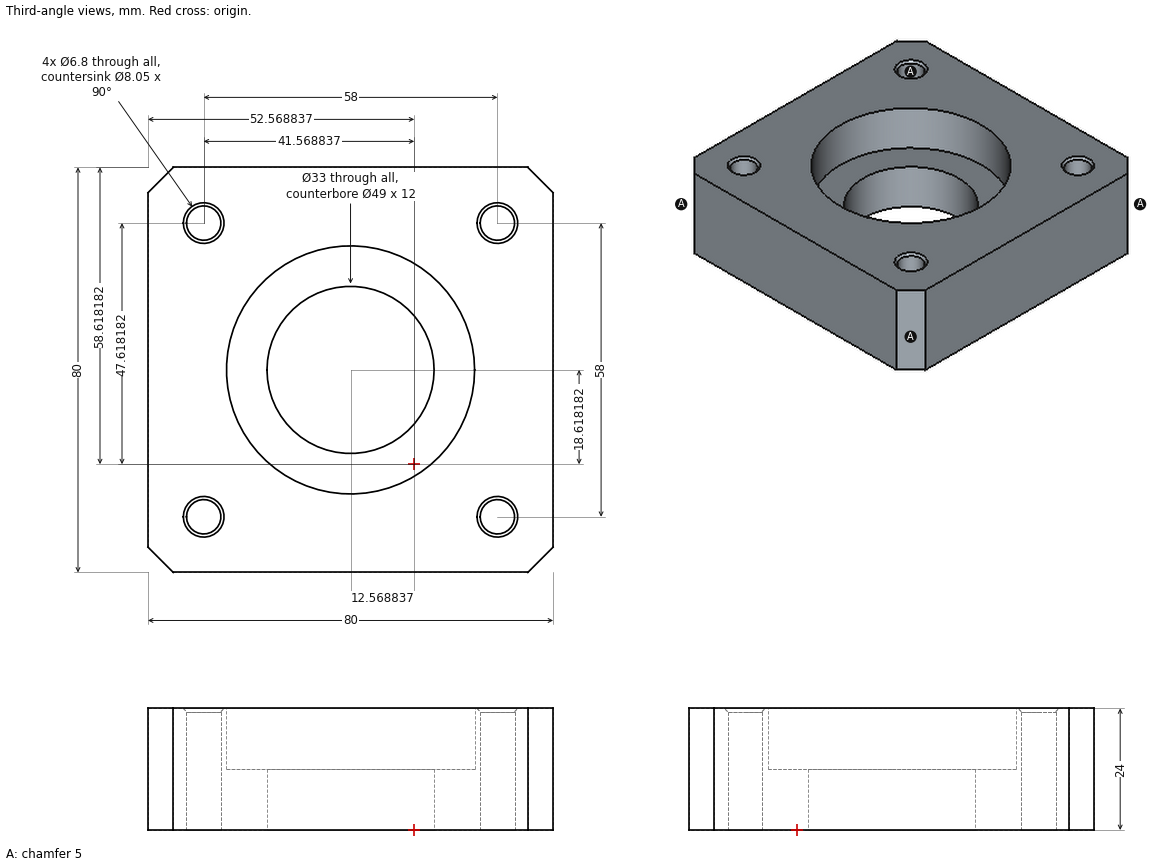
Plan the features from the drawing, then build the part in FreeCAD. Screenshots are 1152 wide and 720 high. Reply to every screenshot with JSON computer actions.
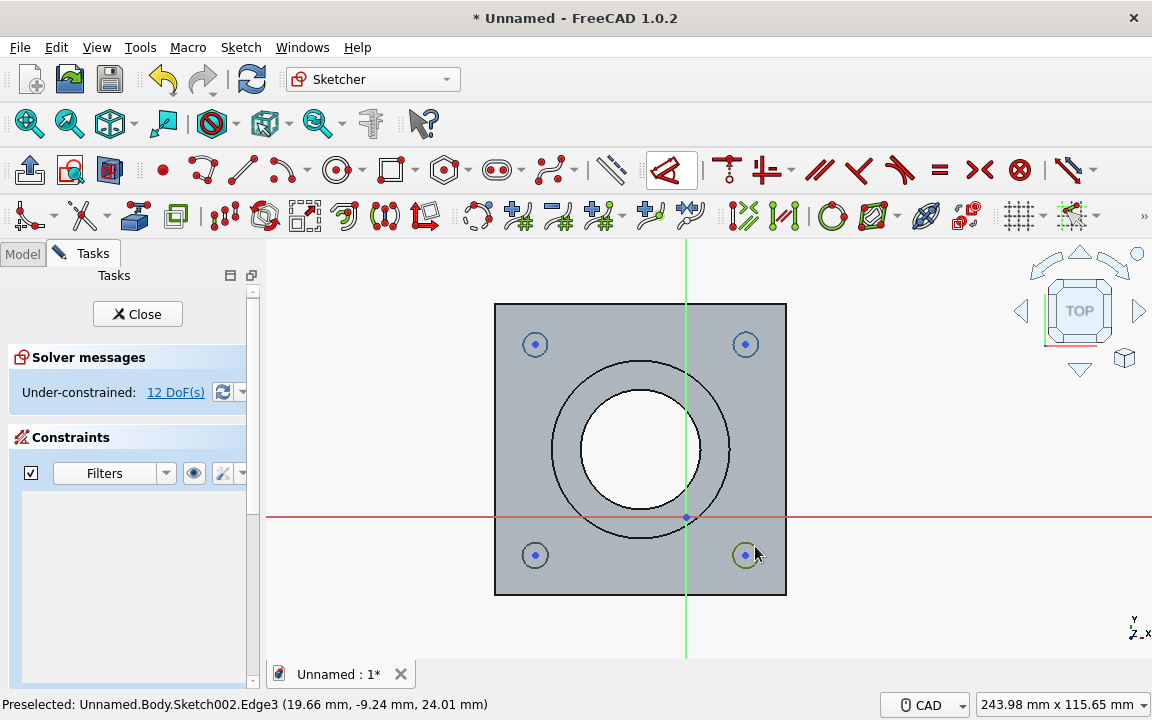
{"action": "left_click", "coordinate": [544, 546]}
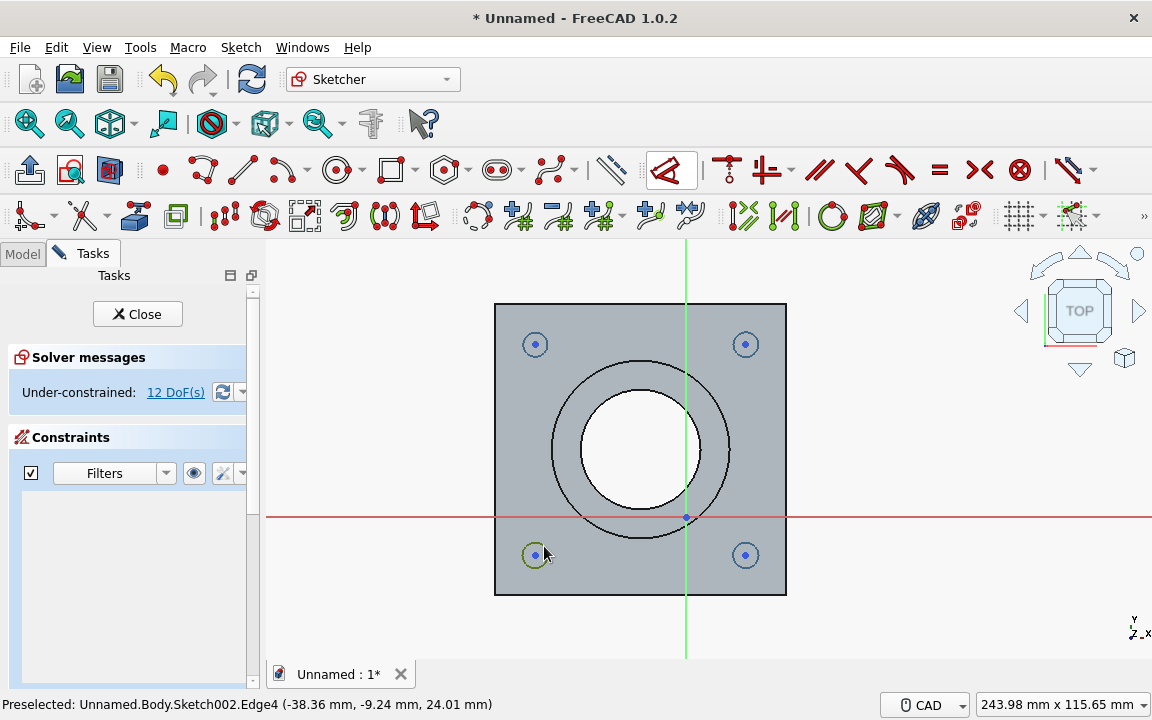
{"action": "key", "text": "e"}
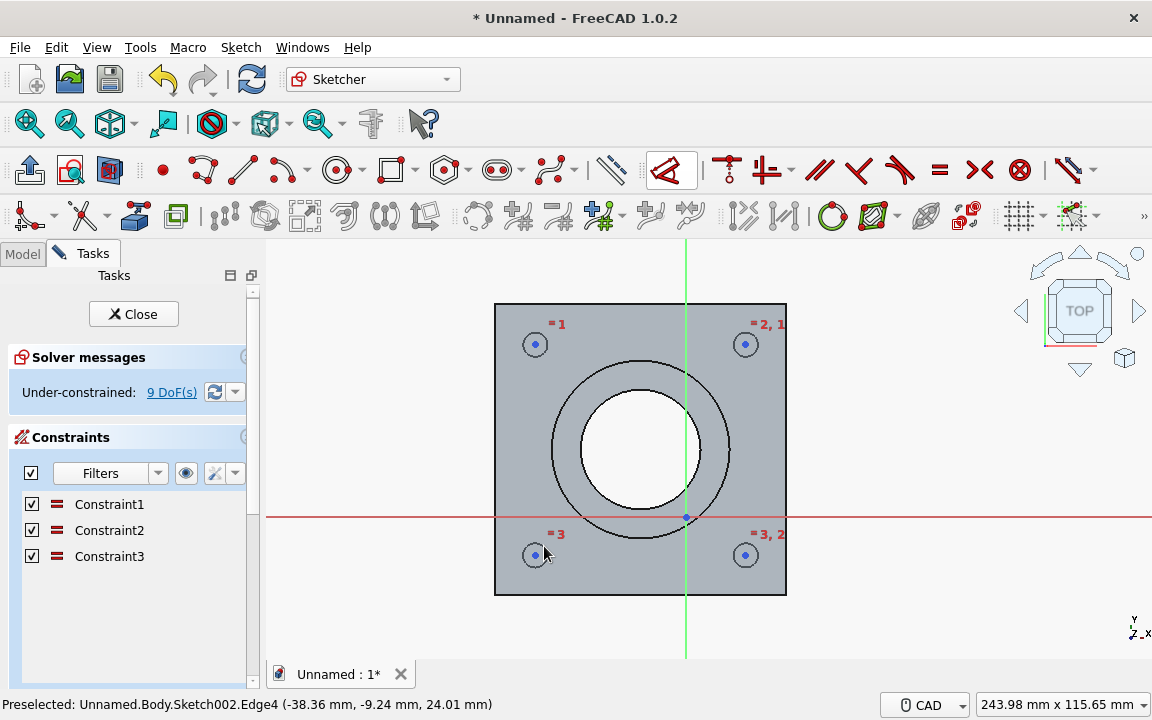
{"action": "scroll", "coordinate": [544, 336], "scroll_direction": "up", "scroll_amount": 3}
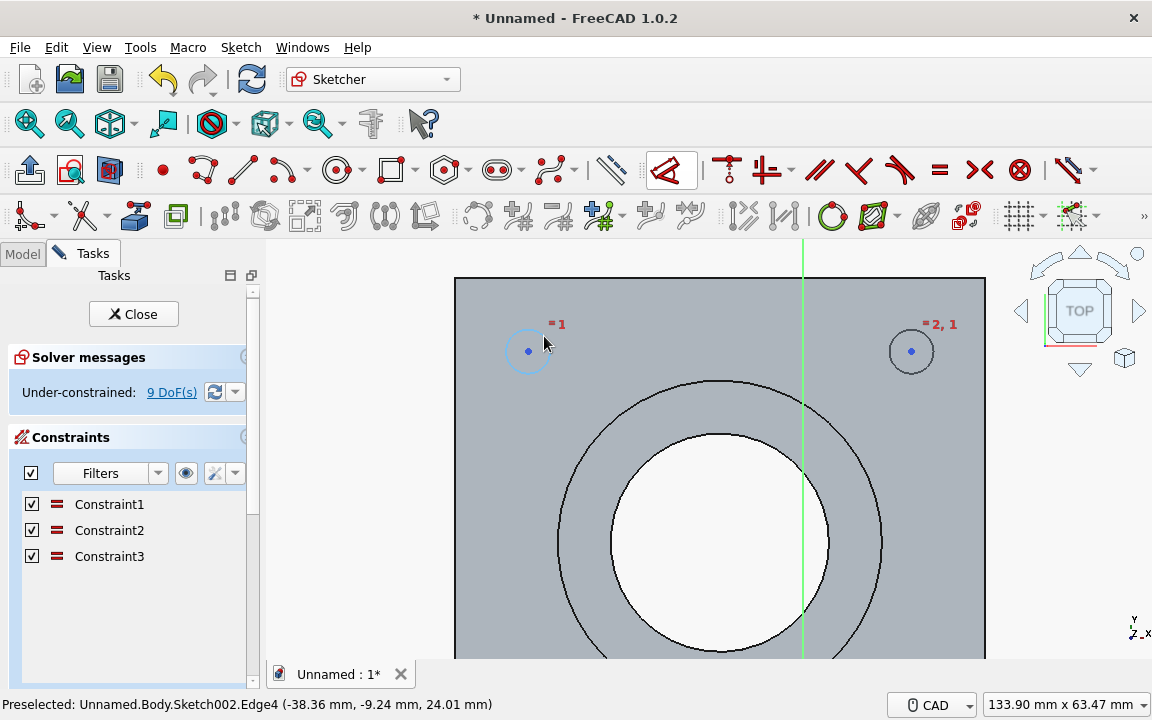
{"action": "left_click", "coordinate": [544, 336]}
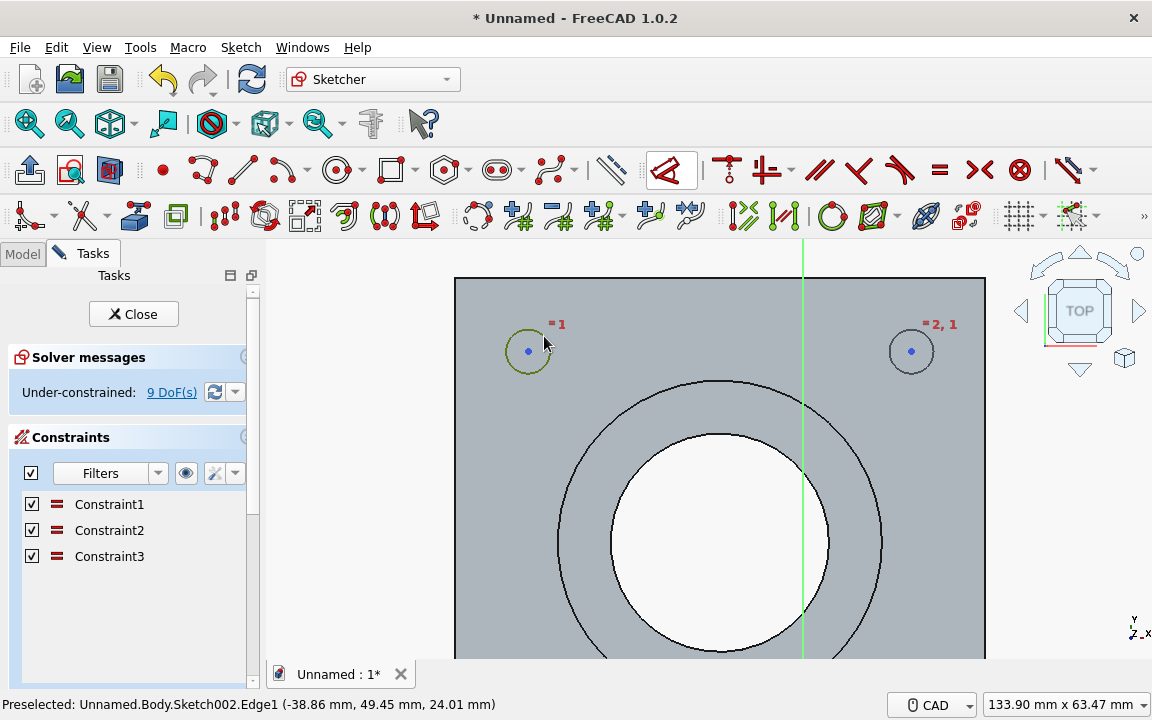
{"action": "key", "text": "k o"}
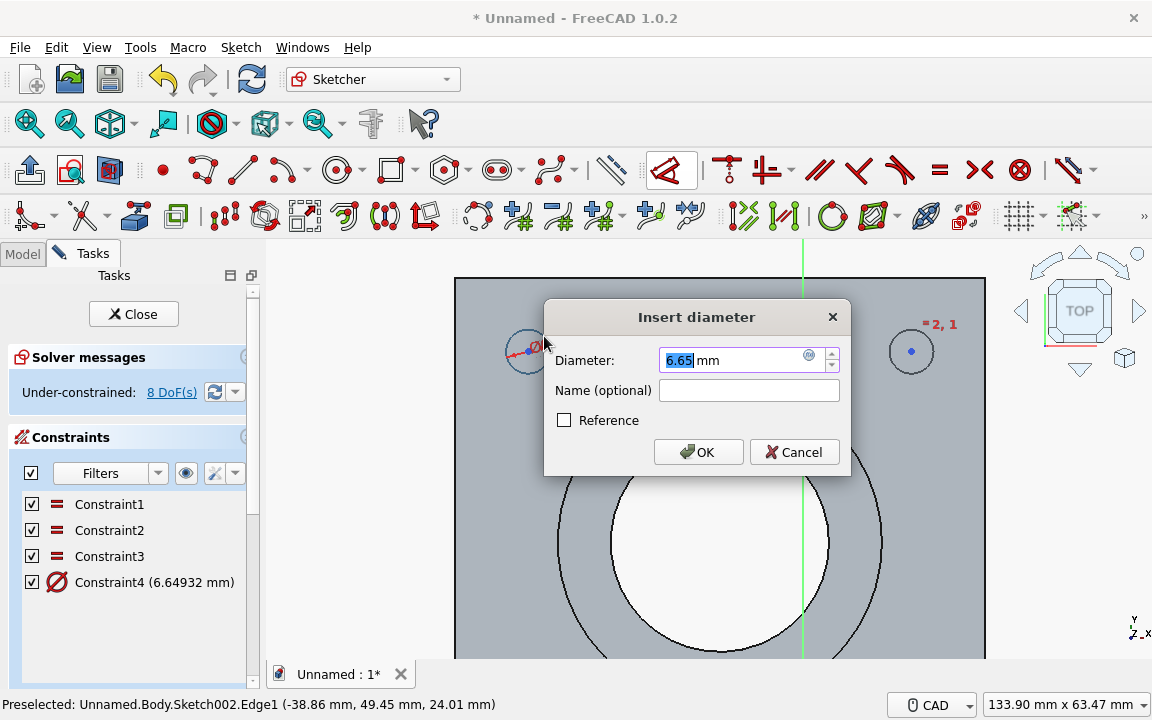
{"action": "type", "text": "6.8"}
{"action": "key", "text": "Return"}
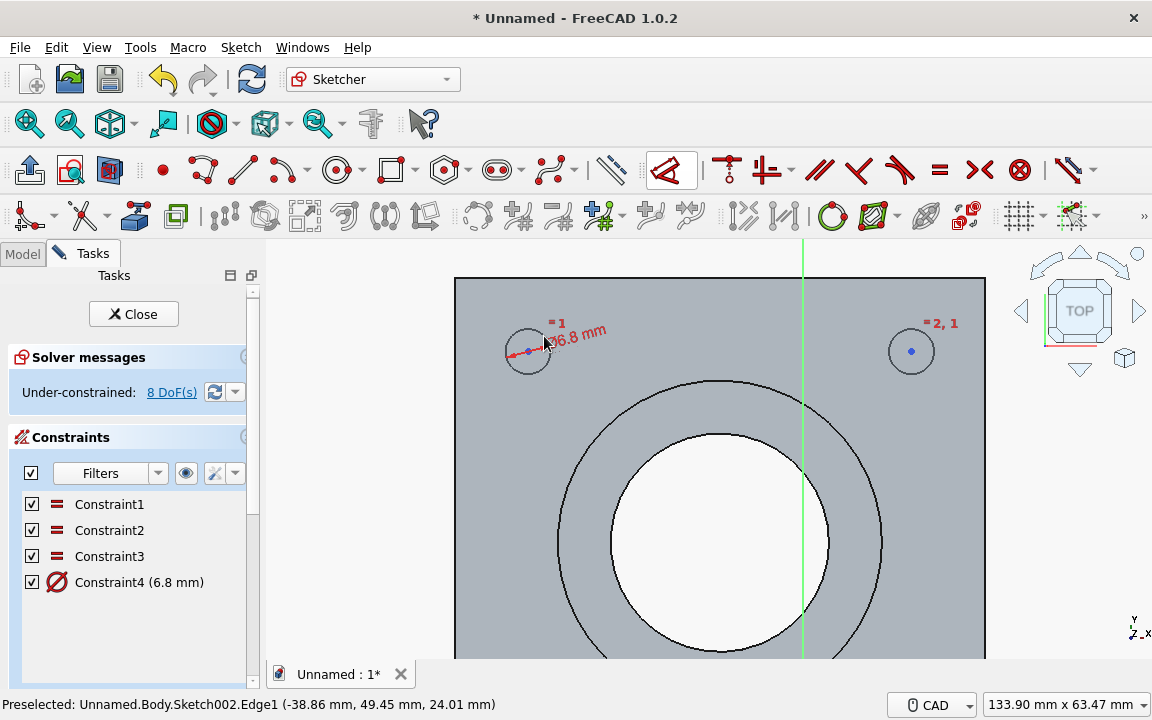
{"action": "left_click", "coordinate": [528, 352]}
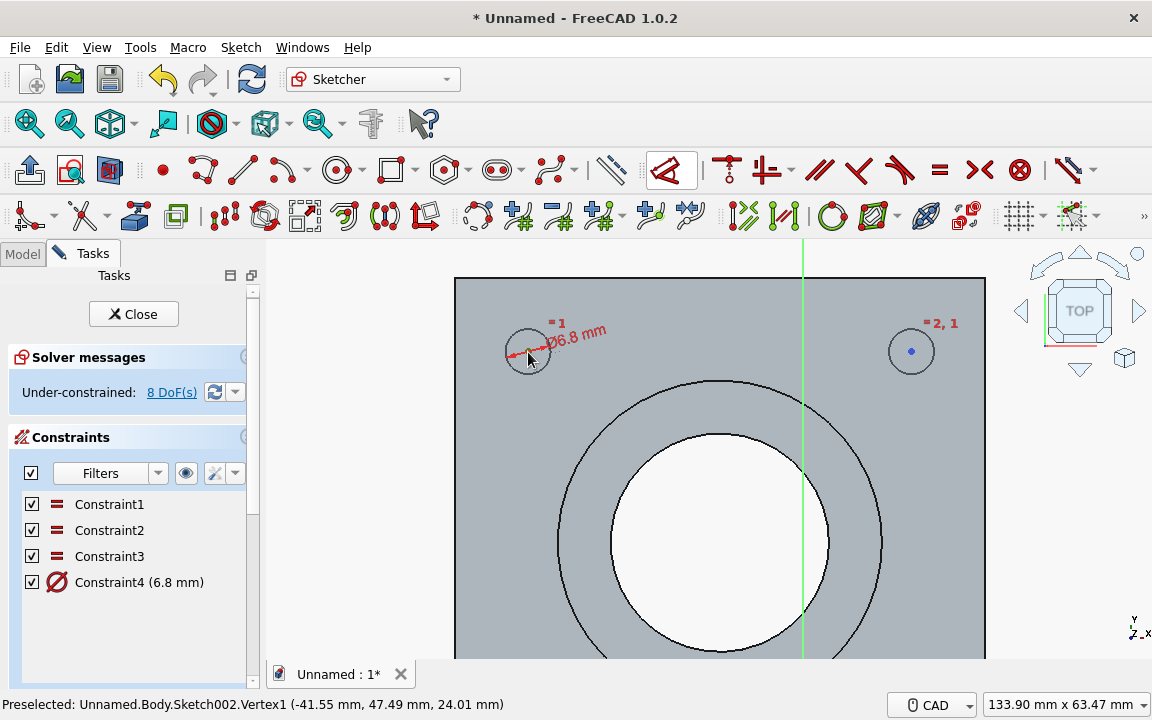
{"action": "left_click", "coordinate": [912, 352]}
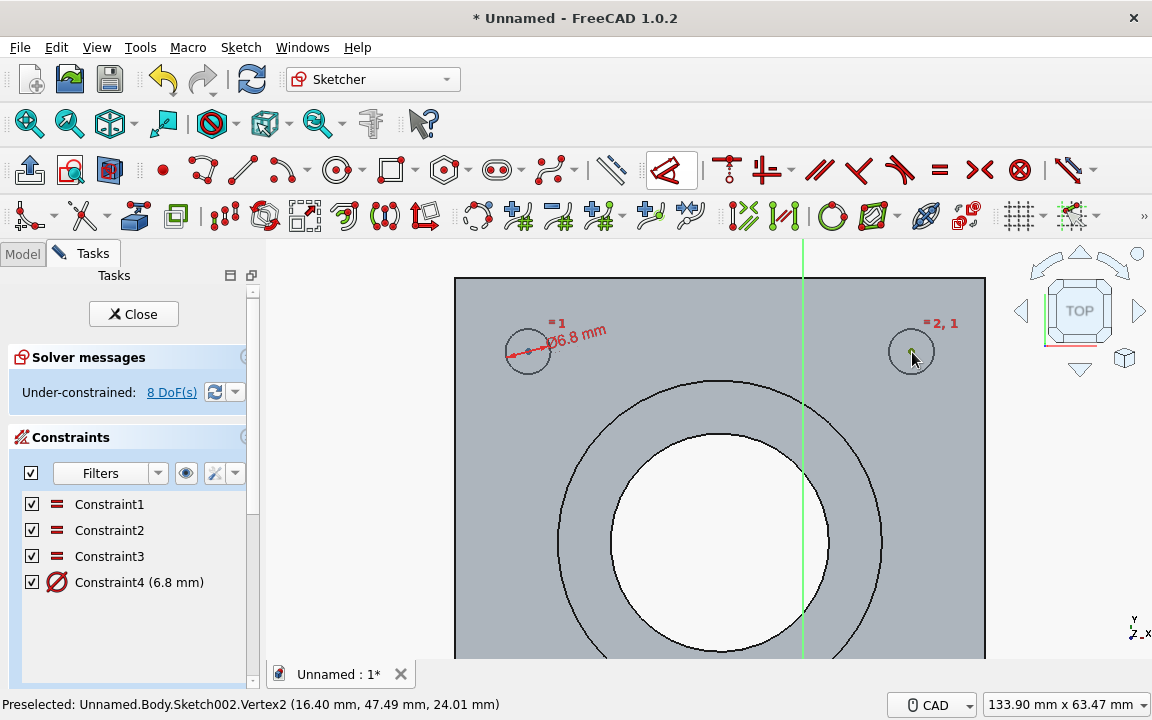
{"action": "left_click", "coordinate": [692, 170]}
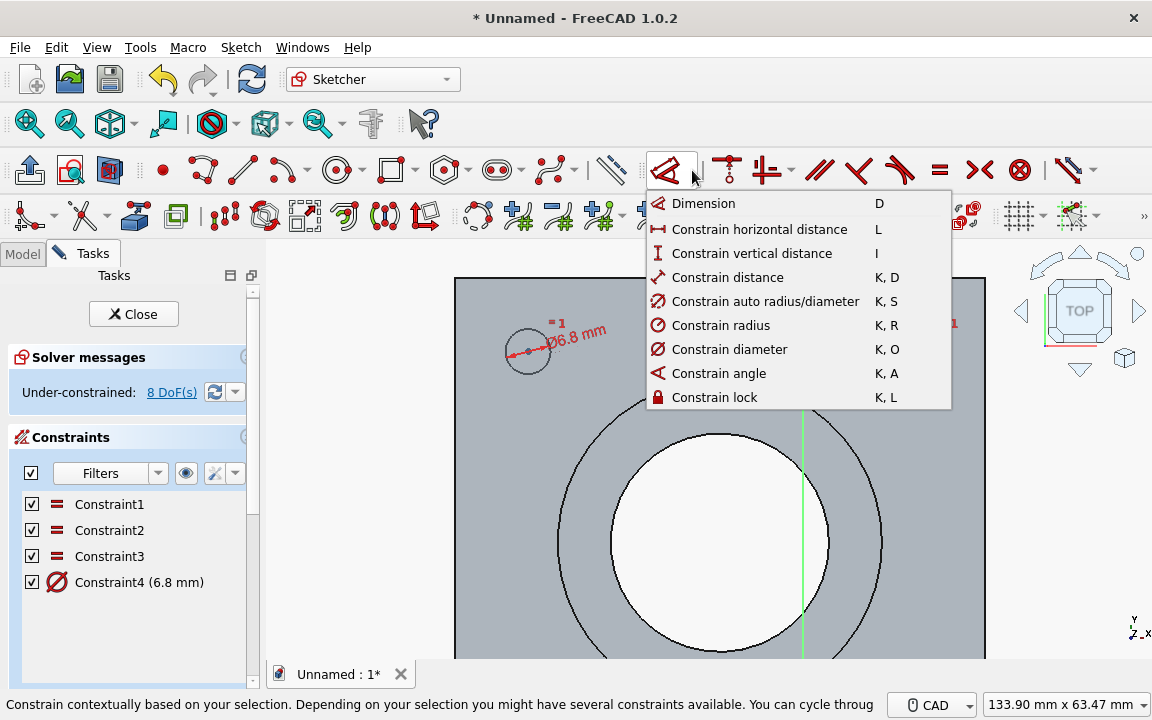
{"action": "left_click", "coordinate": [799, 229]}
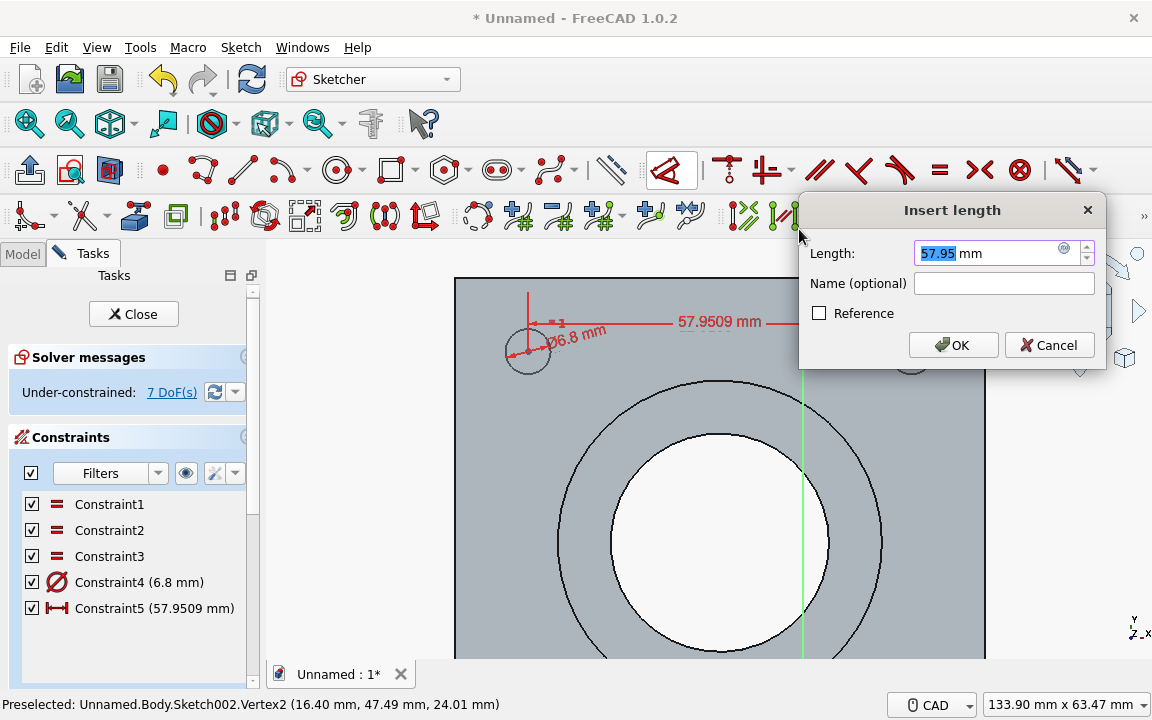
{"action": "type", "text": "58"}
{"action": "key", "text": "Return"}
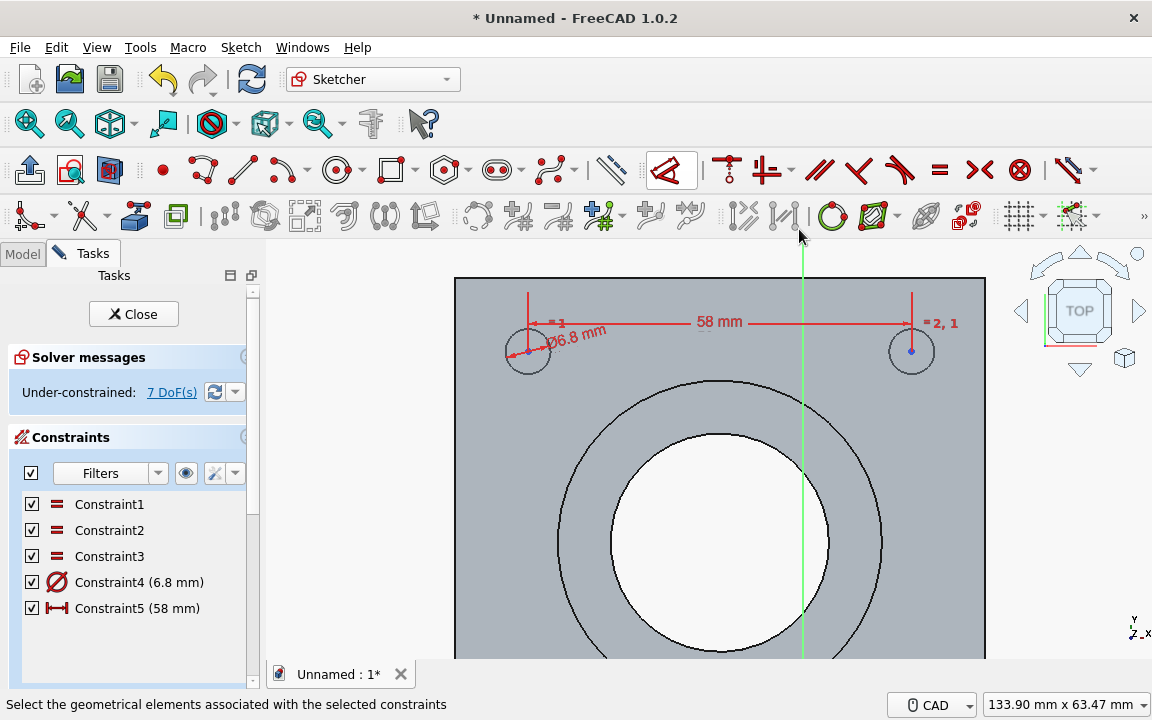
{"action": "left_click", "coordinate": [528, 352]}